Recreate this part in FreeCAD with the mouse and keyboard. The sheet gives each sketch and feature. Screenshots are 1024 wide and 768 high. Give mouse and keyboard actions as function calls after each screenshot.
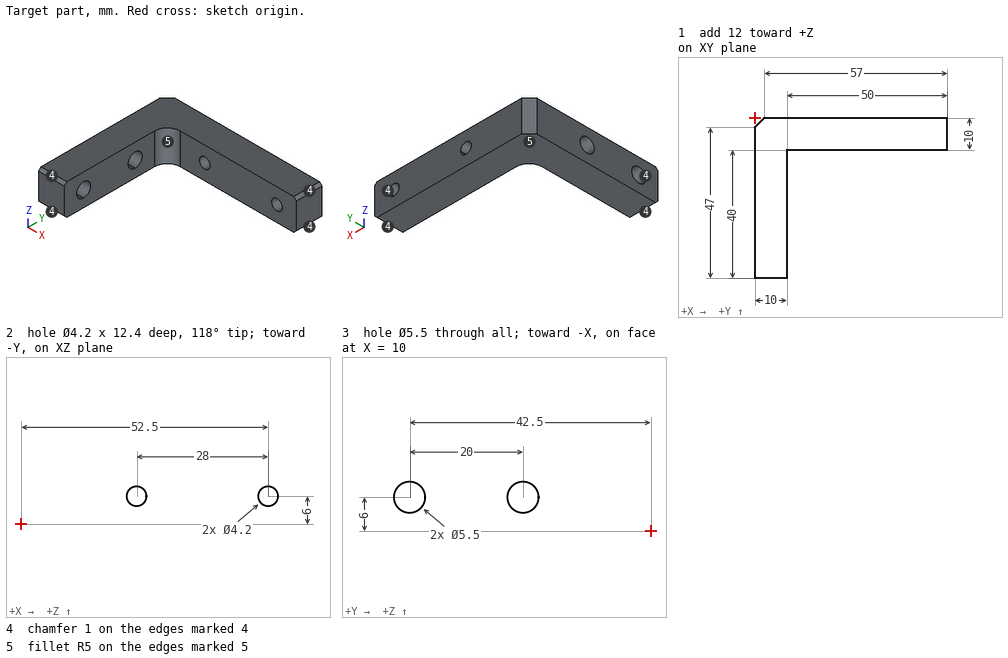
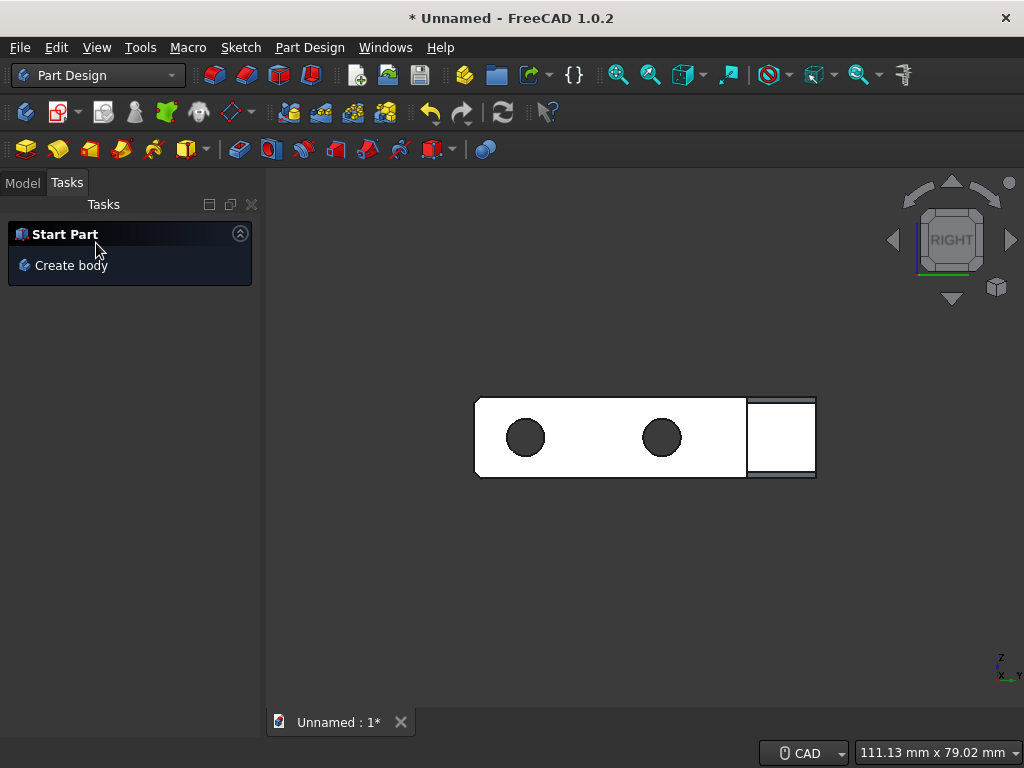
key(0)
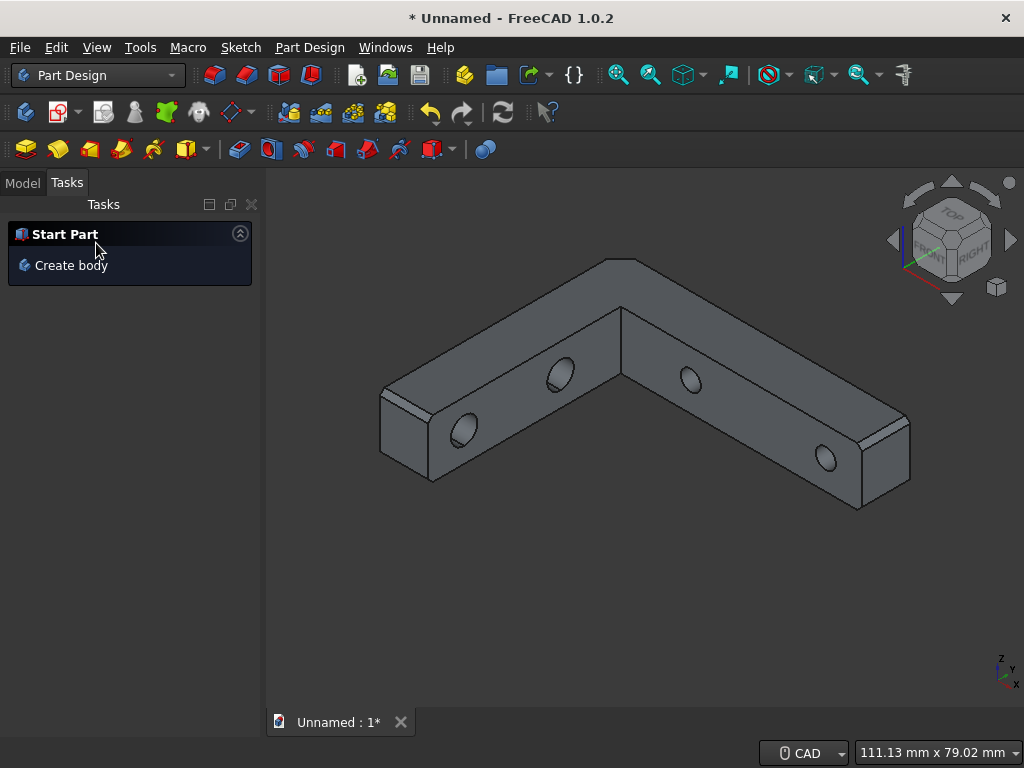
key(2)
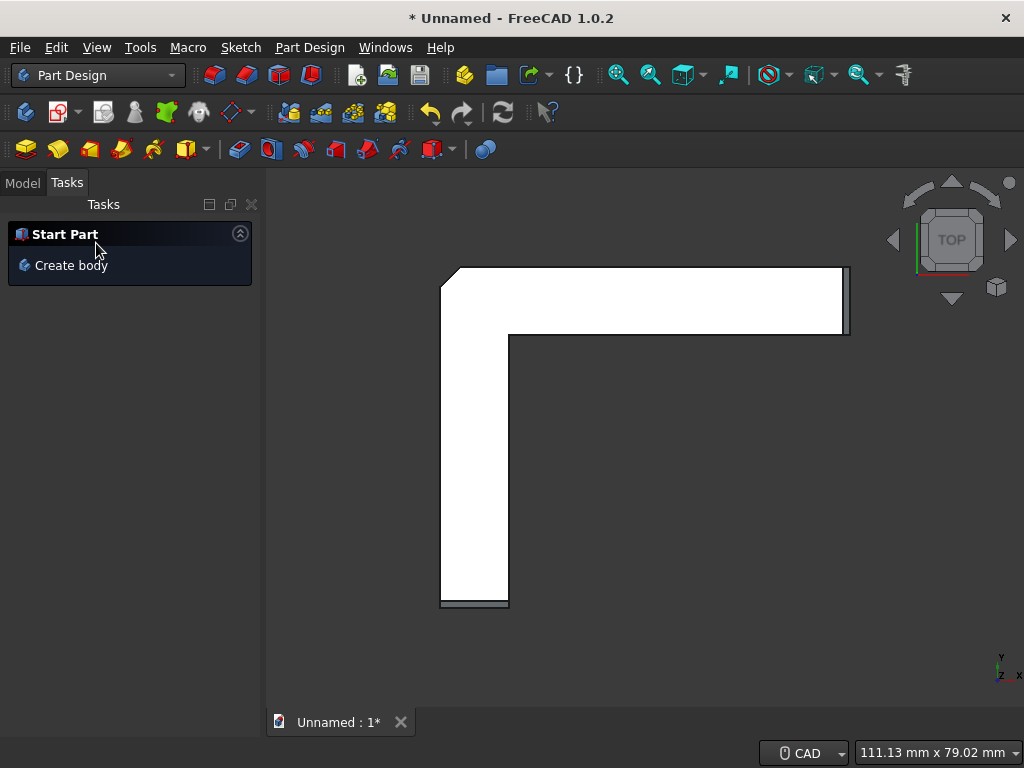
key(1)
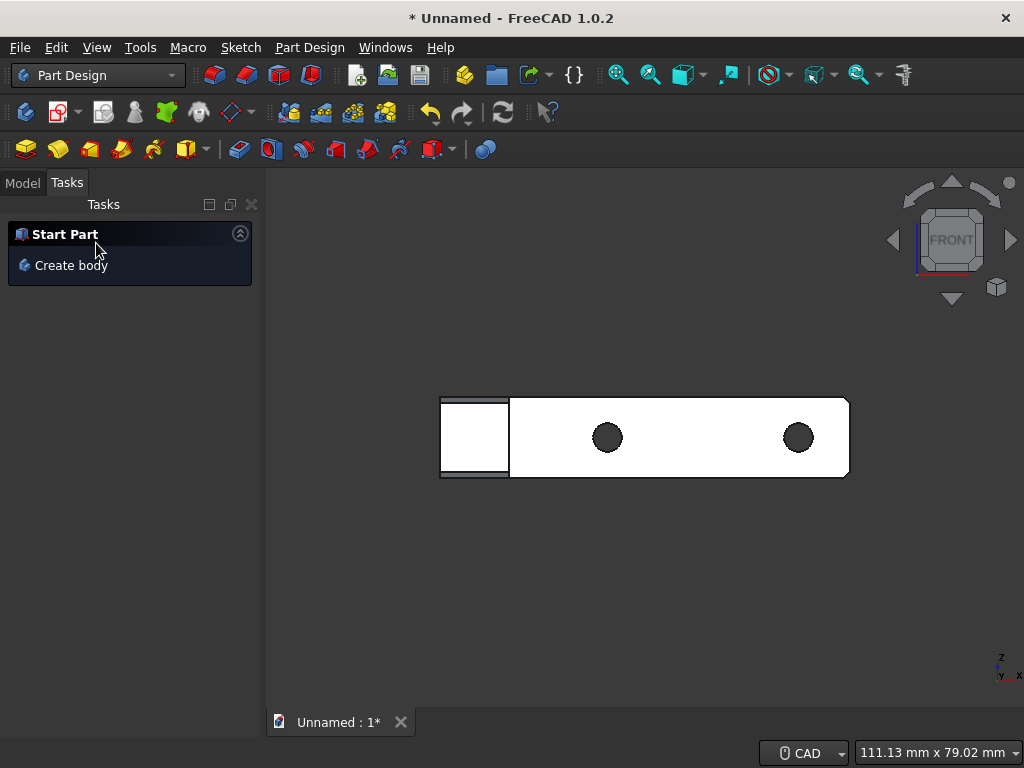
key(3)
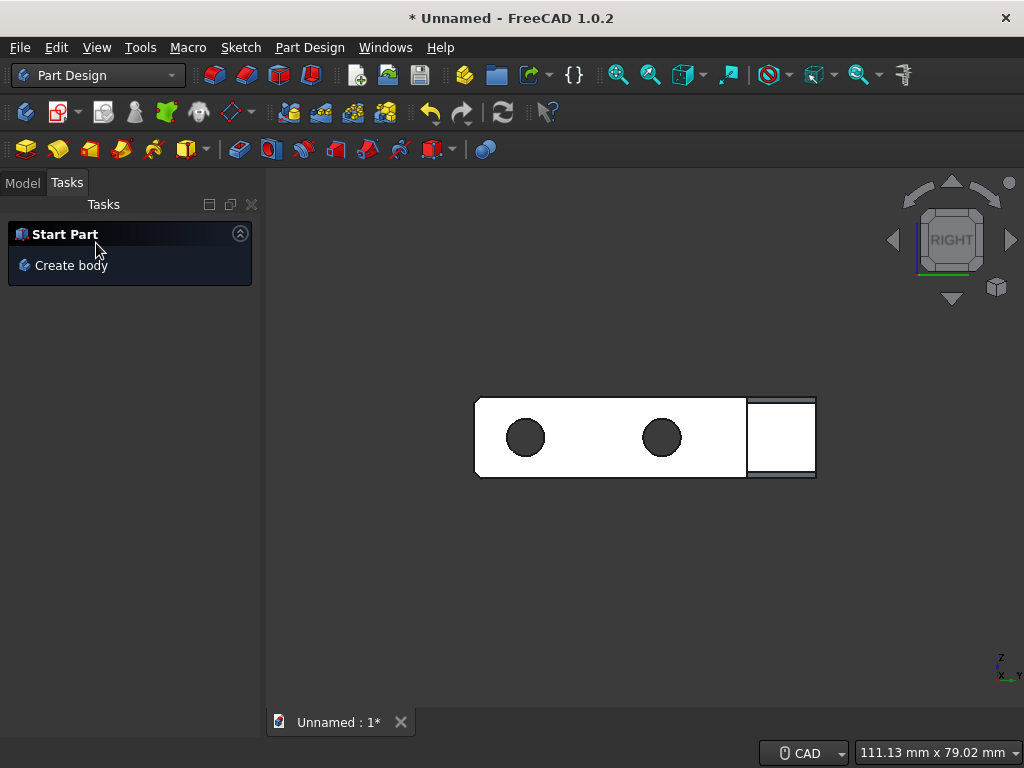
key(5)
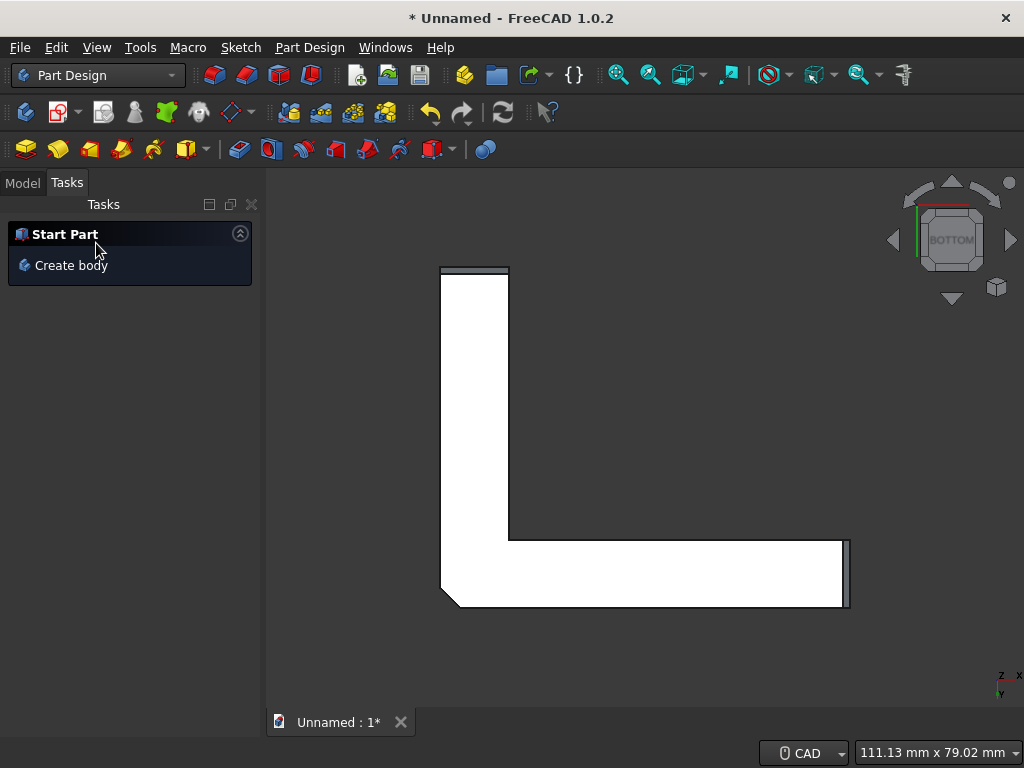
key(4)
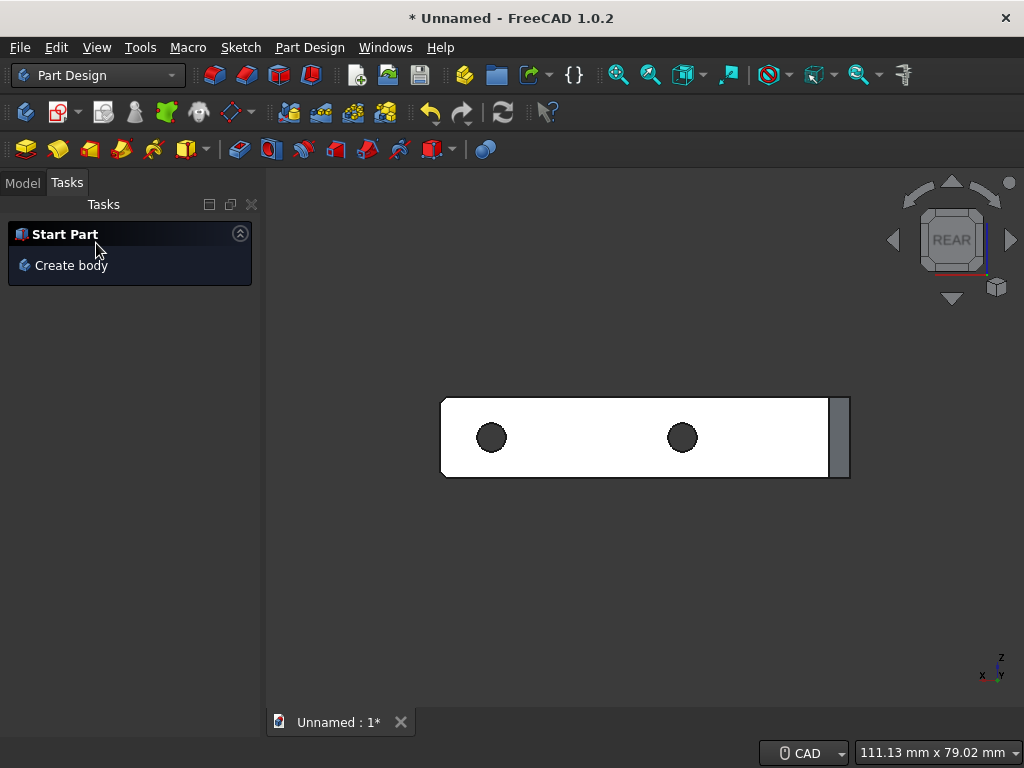
key(6)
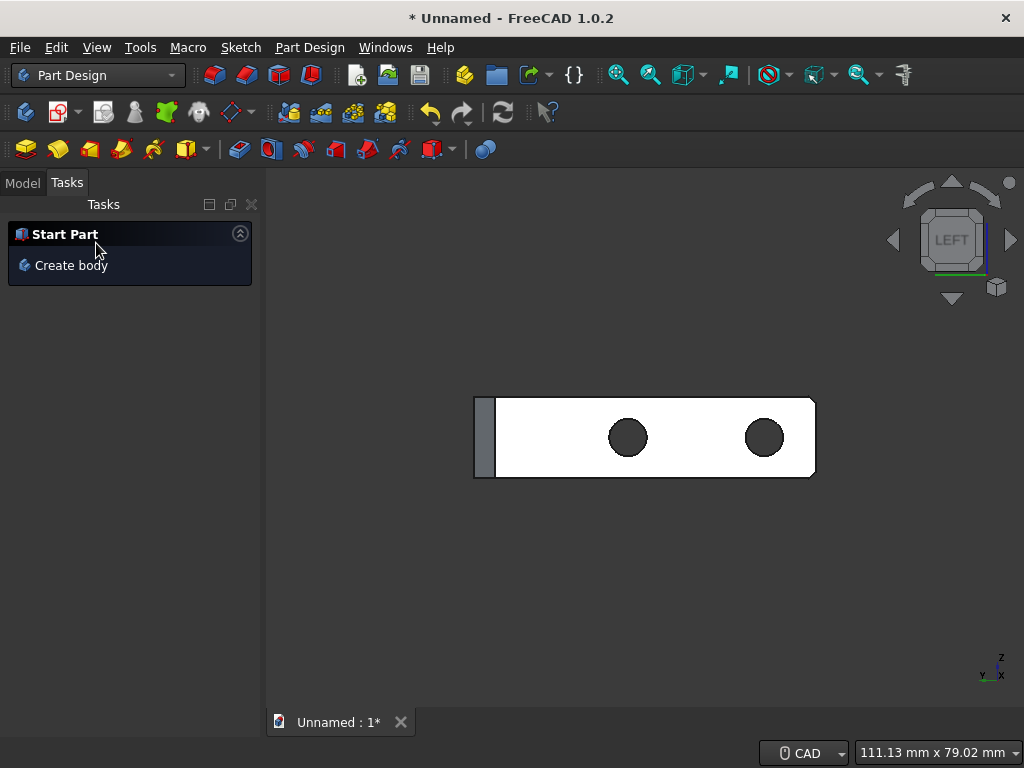
key(v)
key(3)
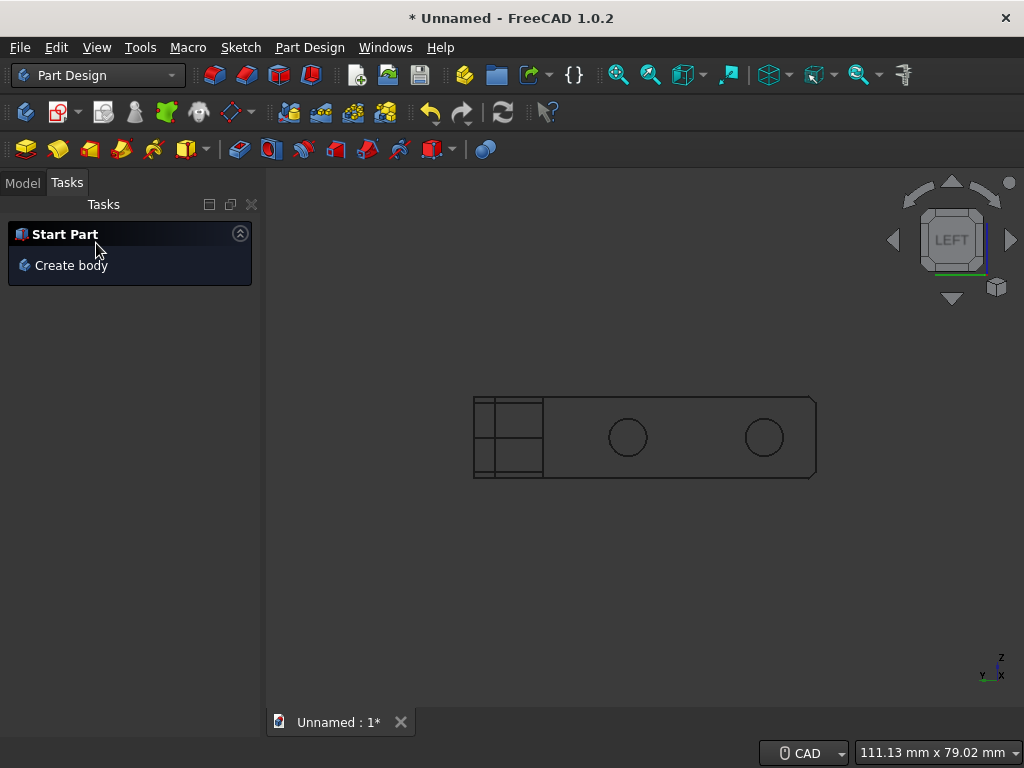
key(0)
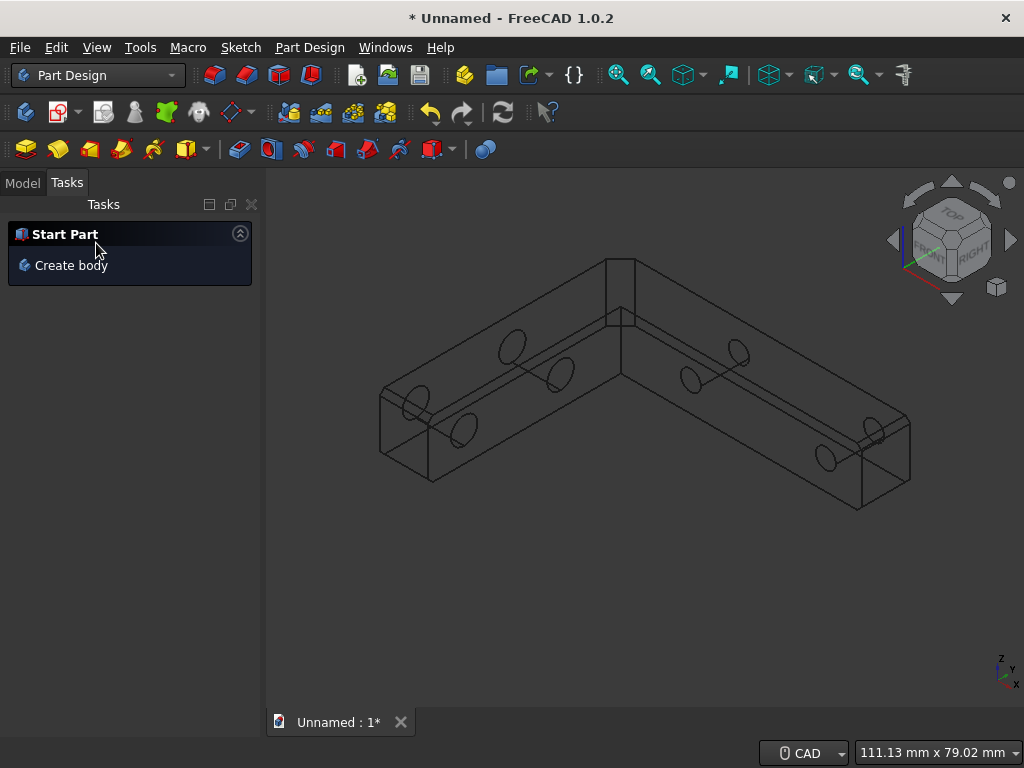
click(621, 339)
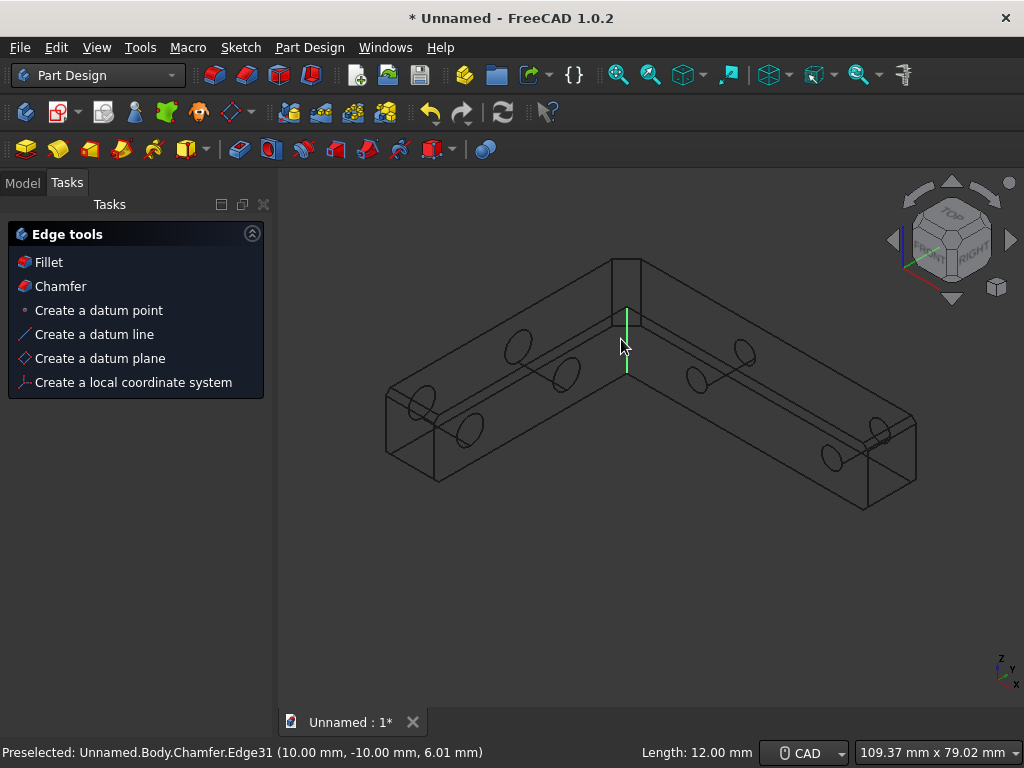
key(v)
key(1)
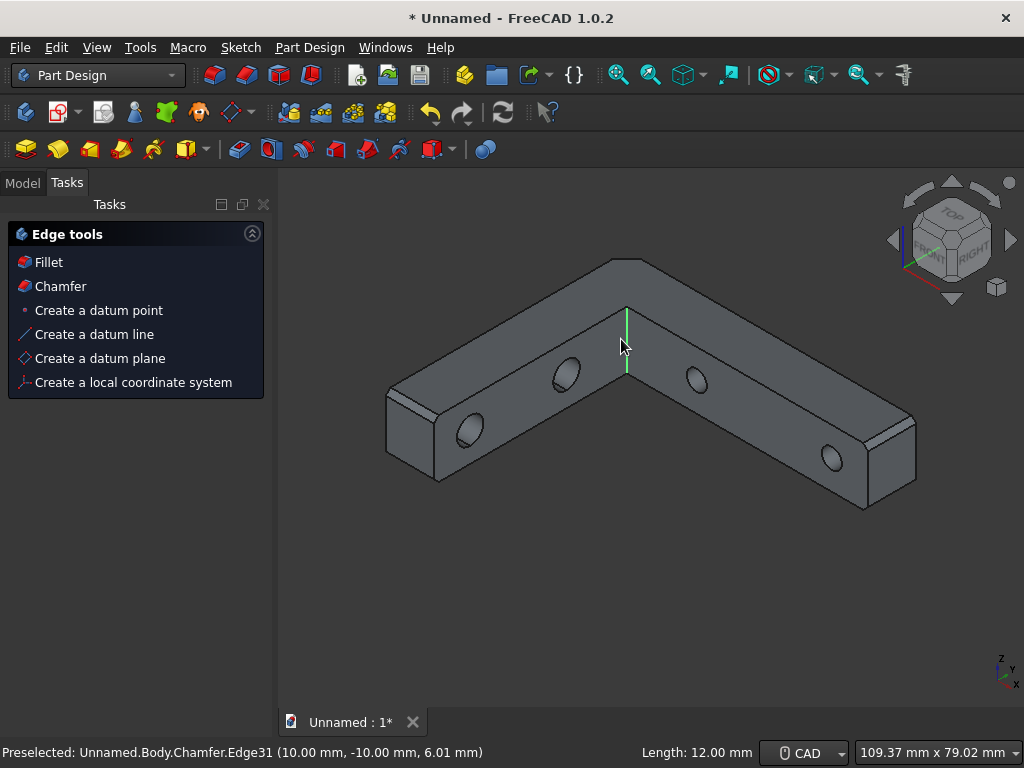
click(216, 76)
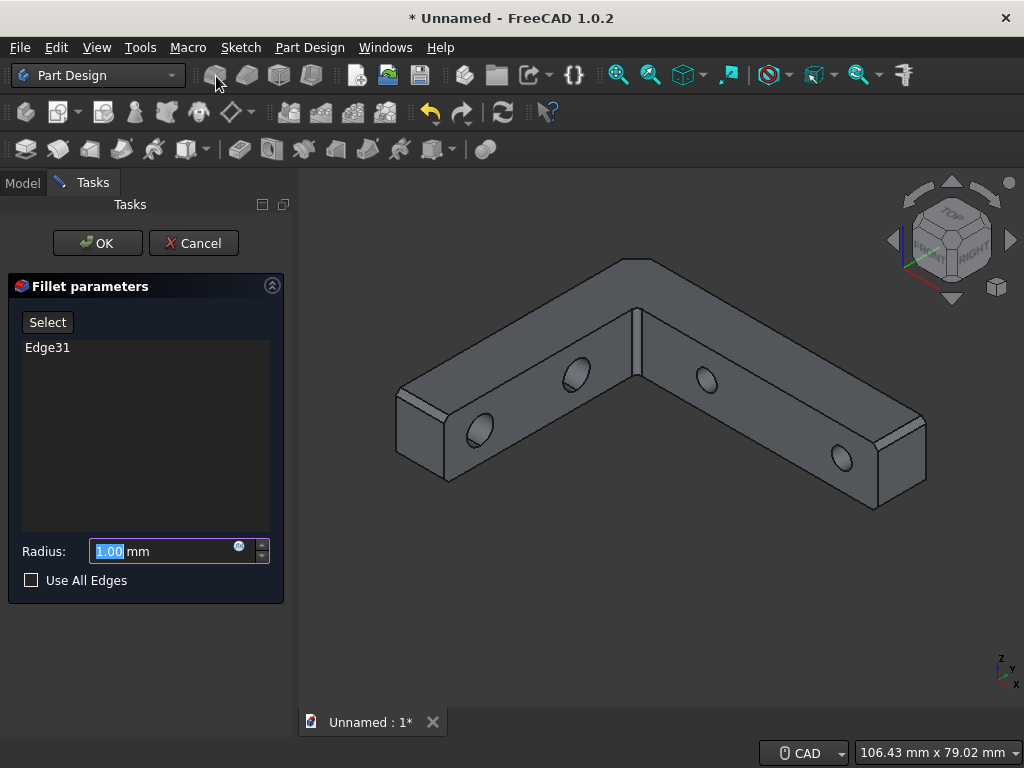
text(5)
key(Tab)